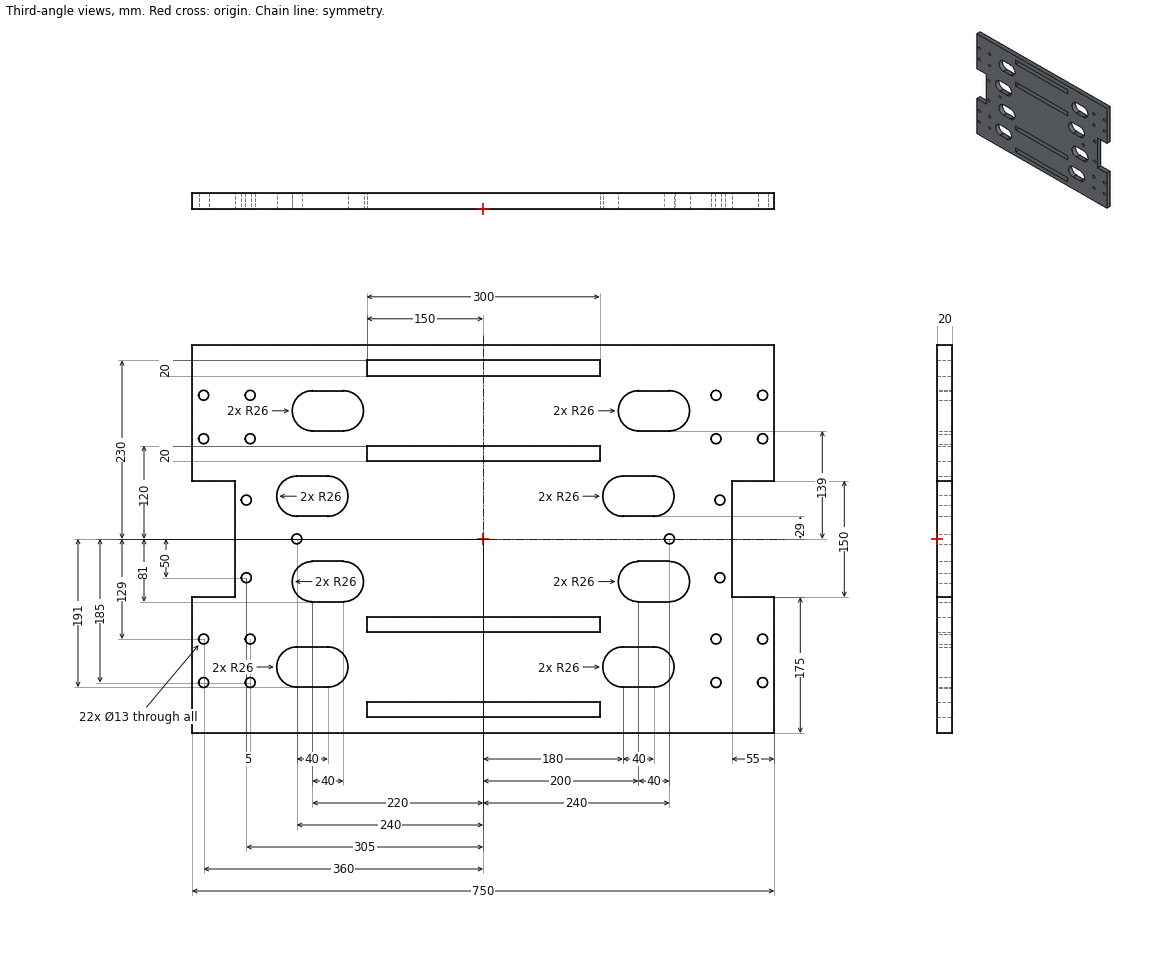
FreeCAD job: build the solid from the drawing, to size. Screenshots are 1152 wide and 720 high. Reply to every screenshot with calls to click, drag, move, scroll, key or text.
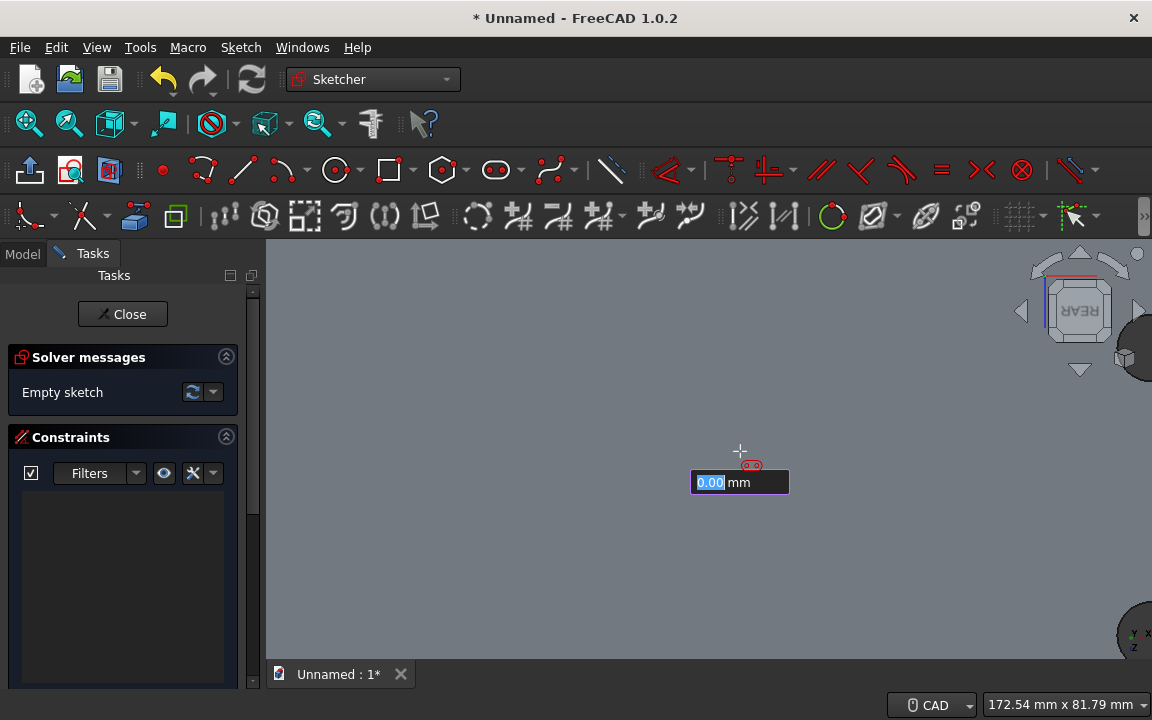
click(637, 317)
key(Escape)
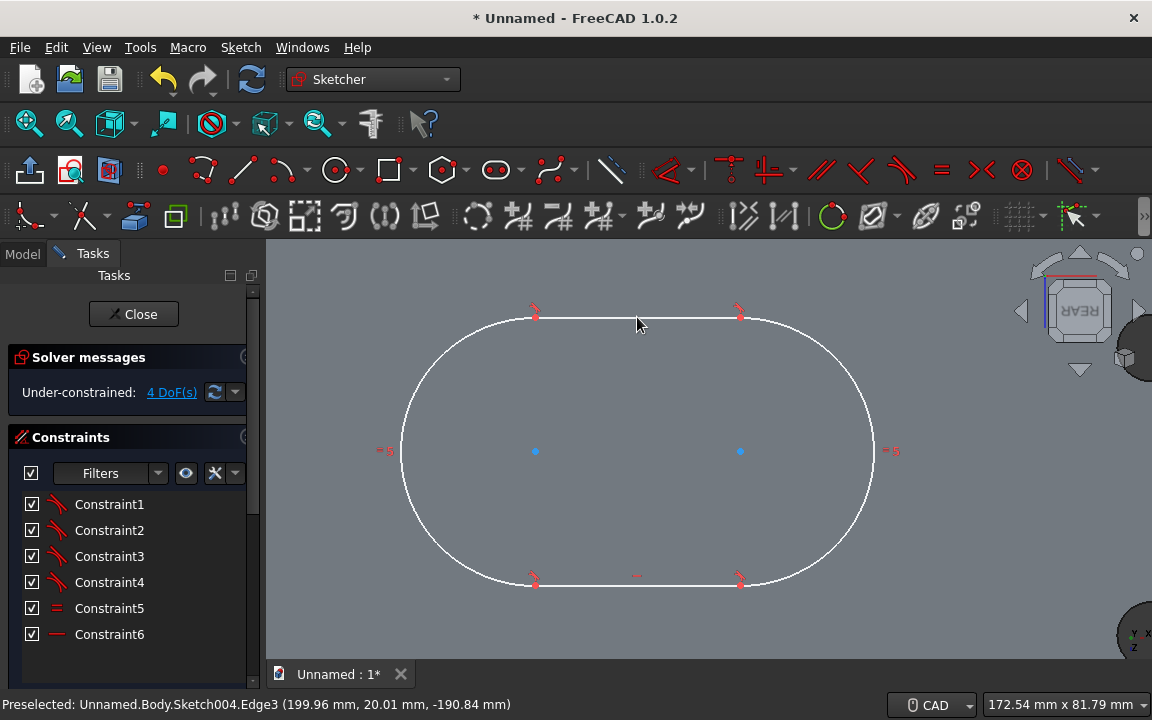
click(666, 170)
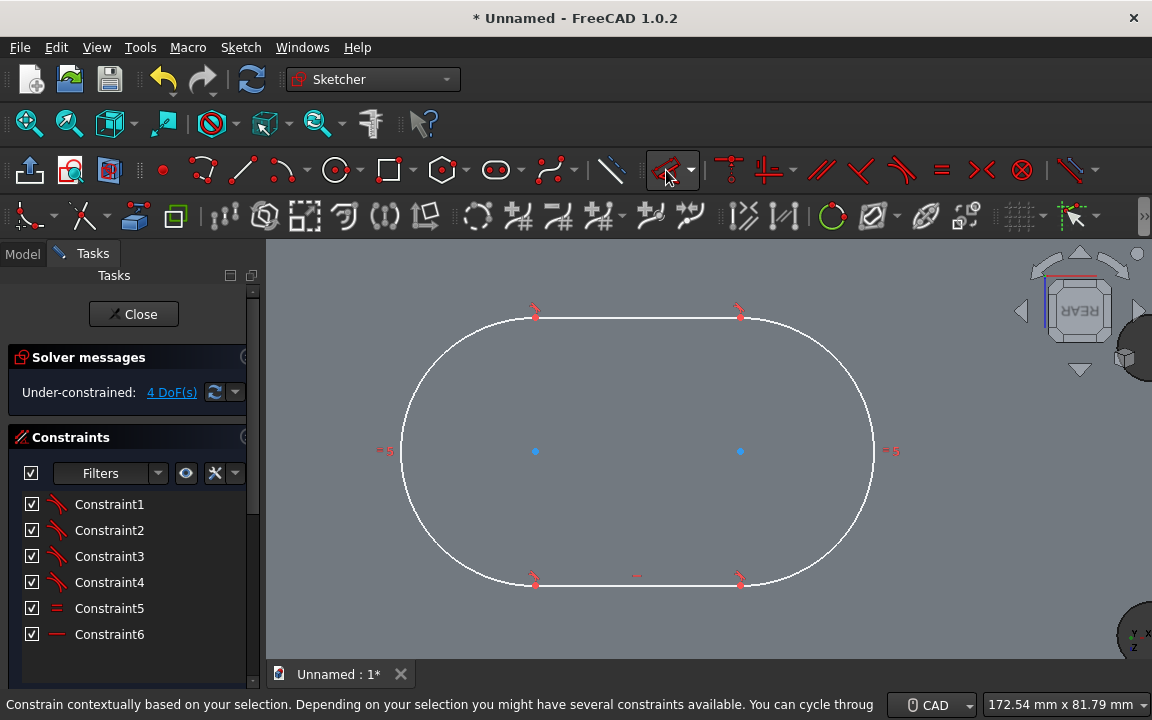
click(427, 373)
click(401, 354)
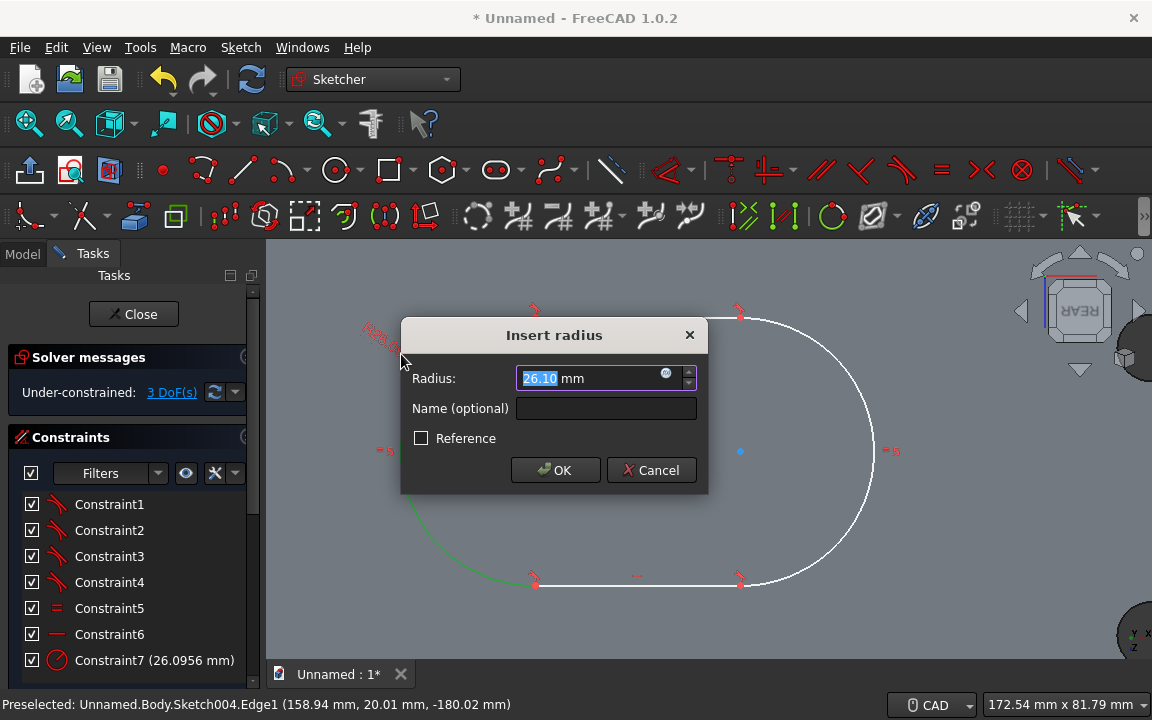
text(26)
key(Return)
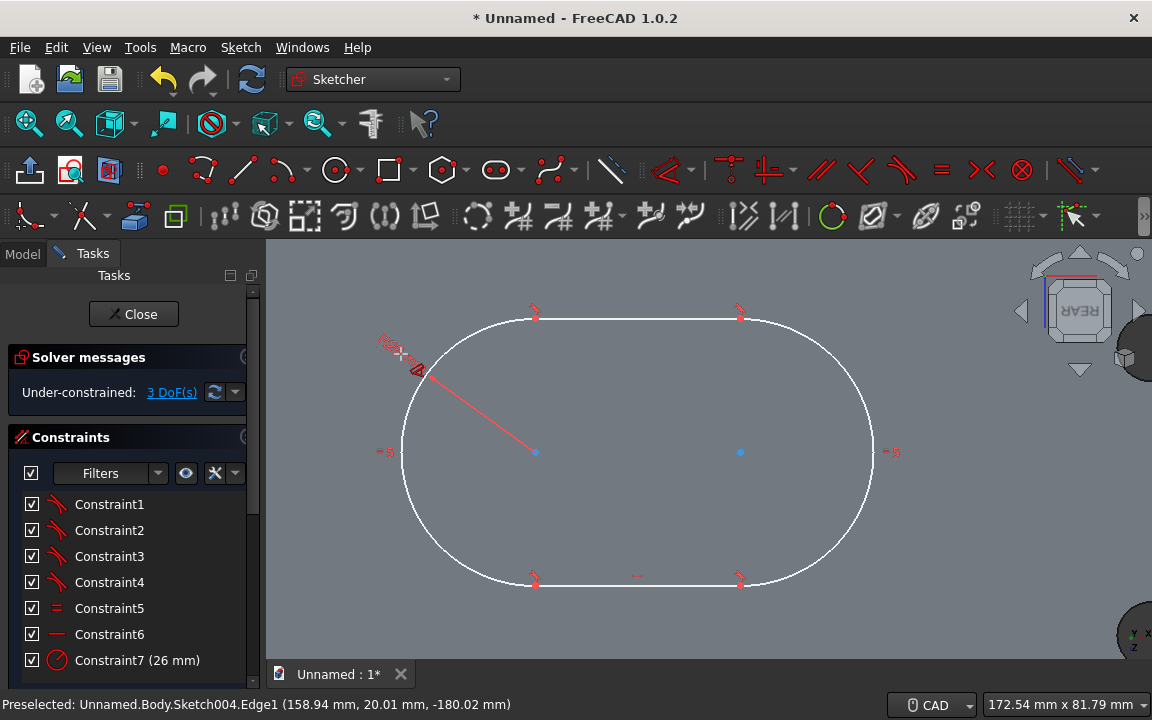
click(597, 319)
click(638, 285)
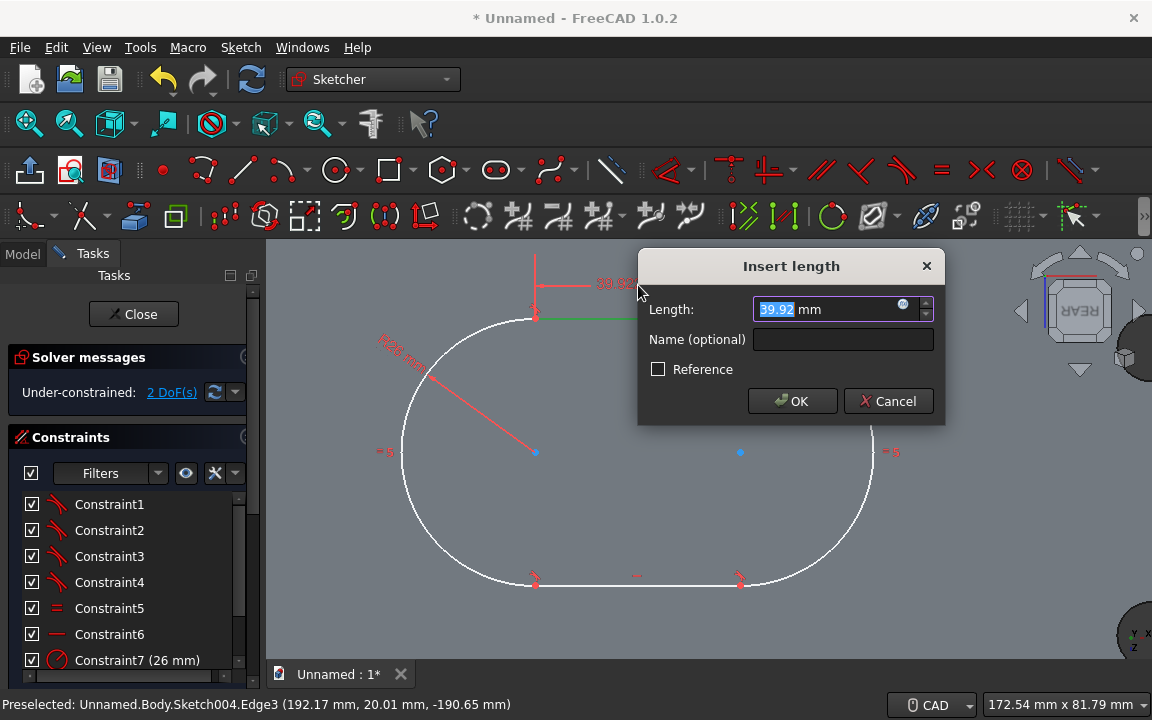
text(40)
key(Return)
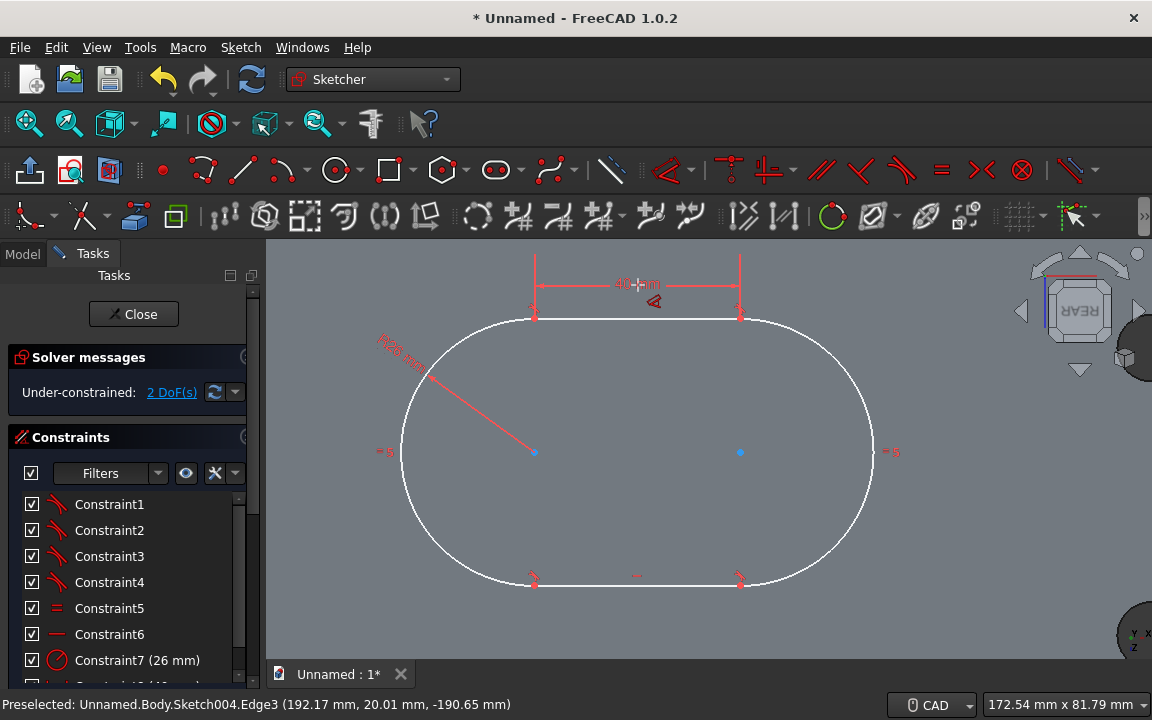
click(535, 319)
click(414, 285)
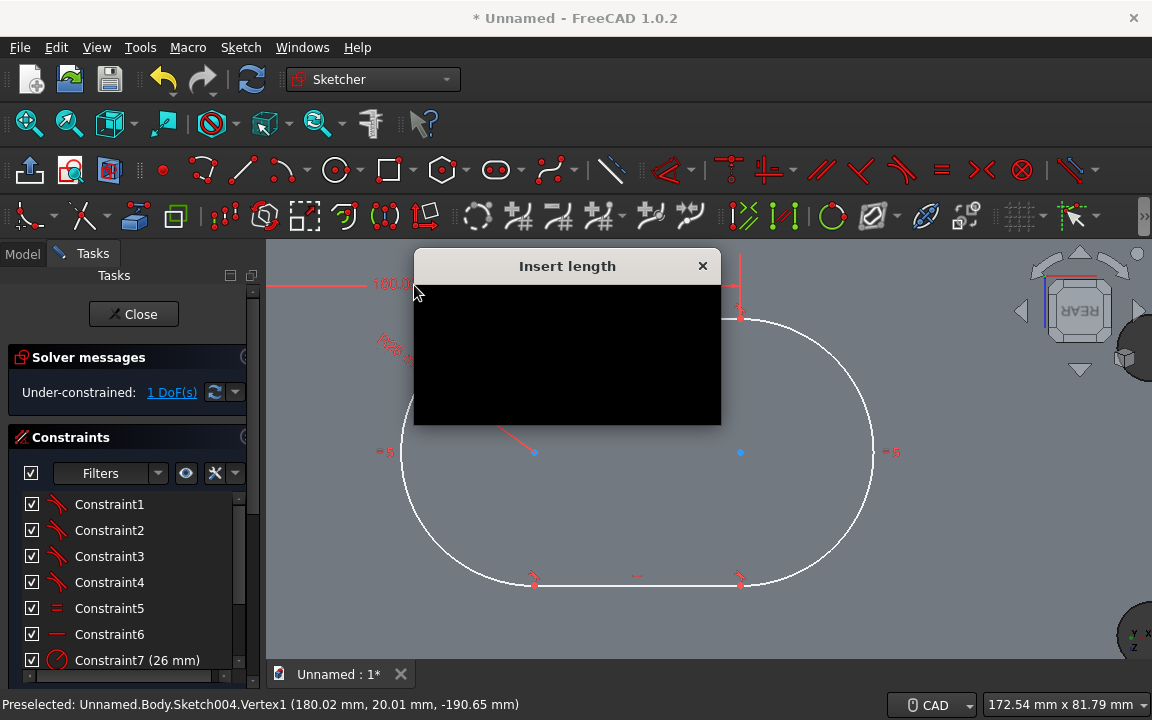
text(180)
key(Return)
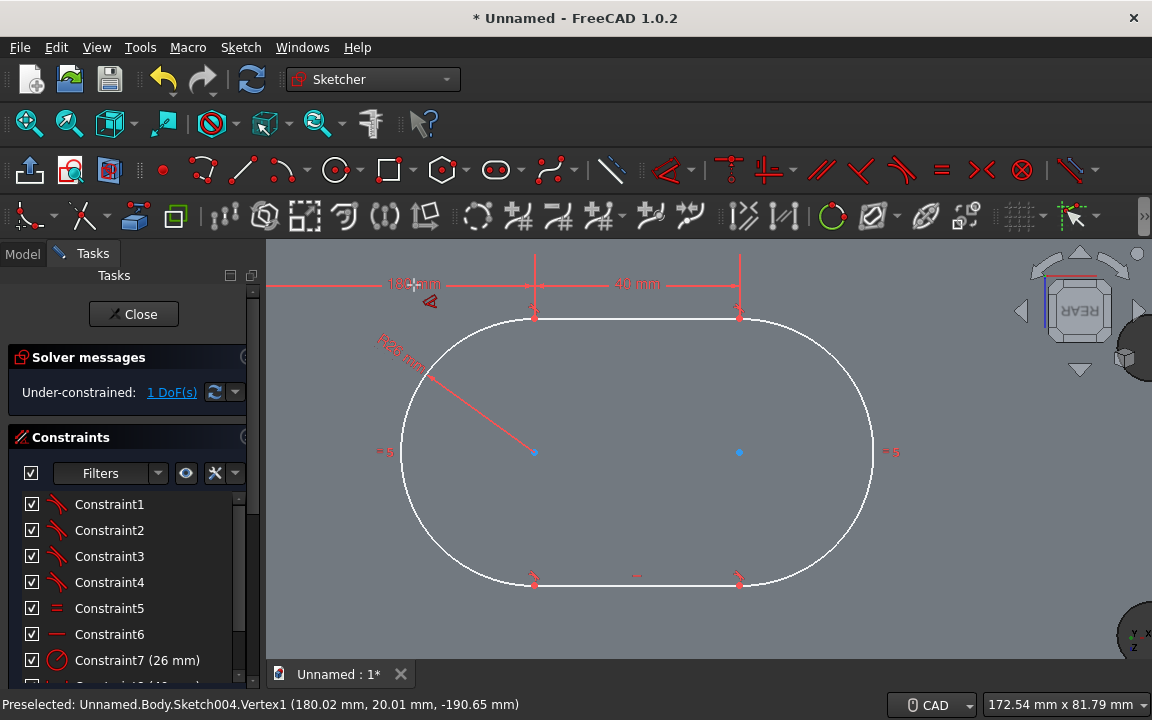
click(535, 319)
click(569, 475)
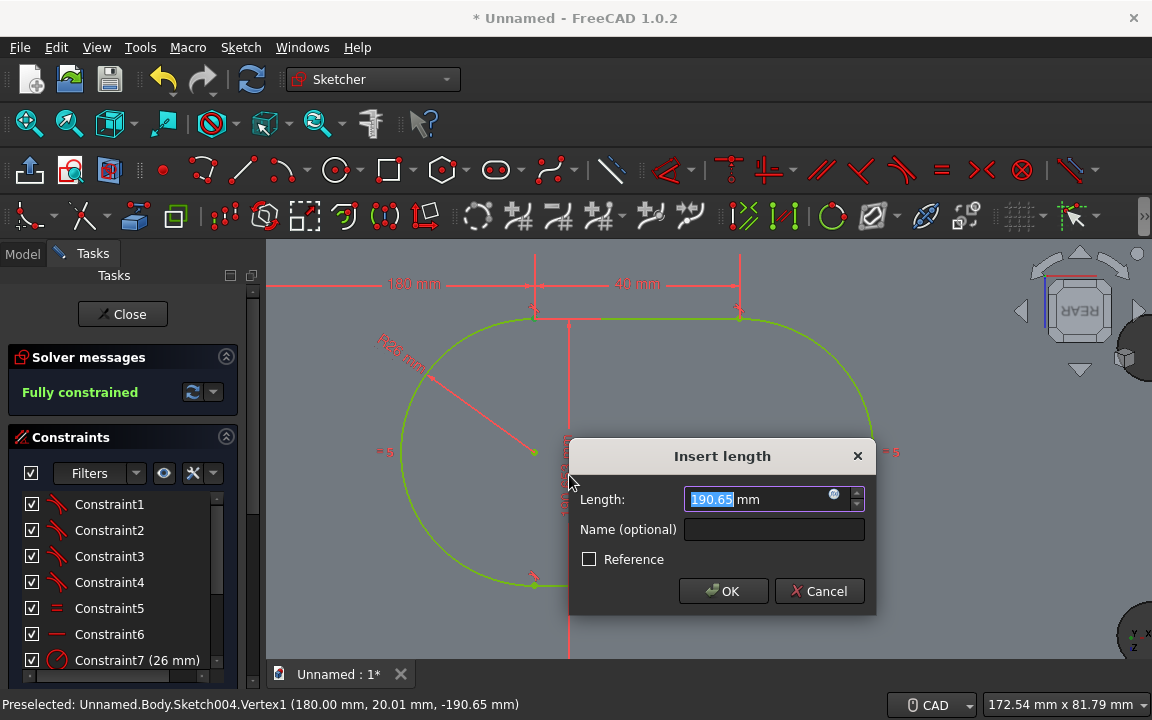
text(191)
key(Return)
key(Escape)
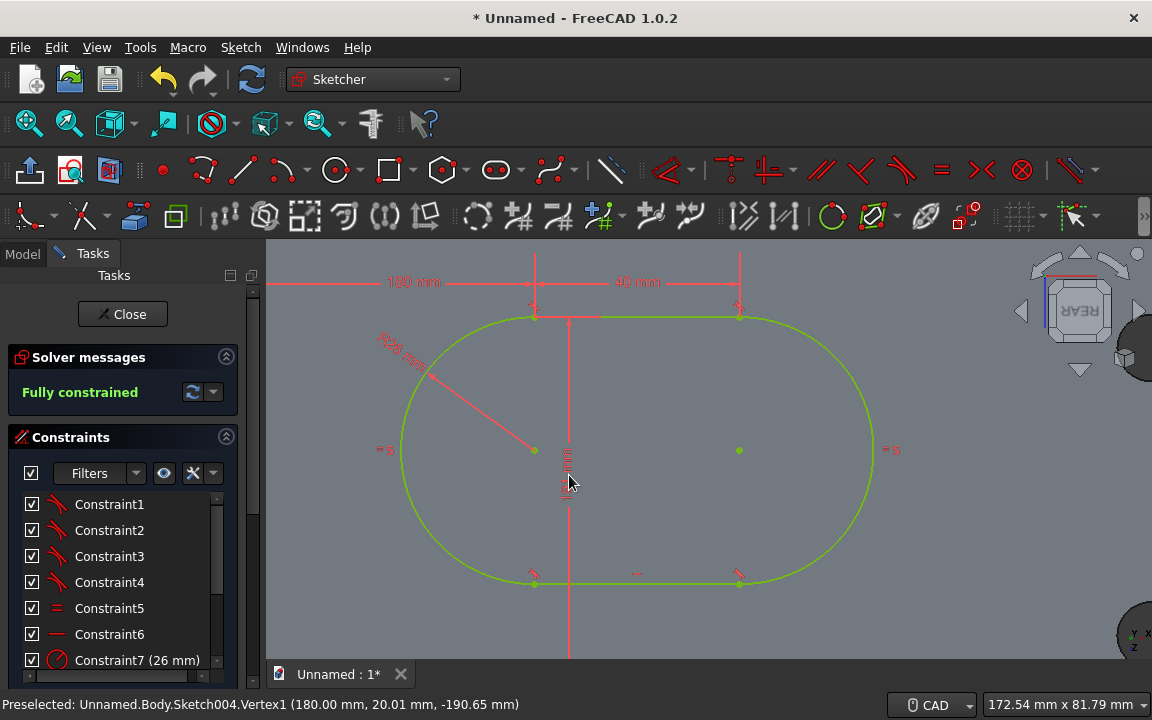
click(123, 314)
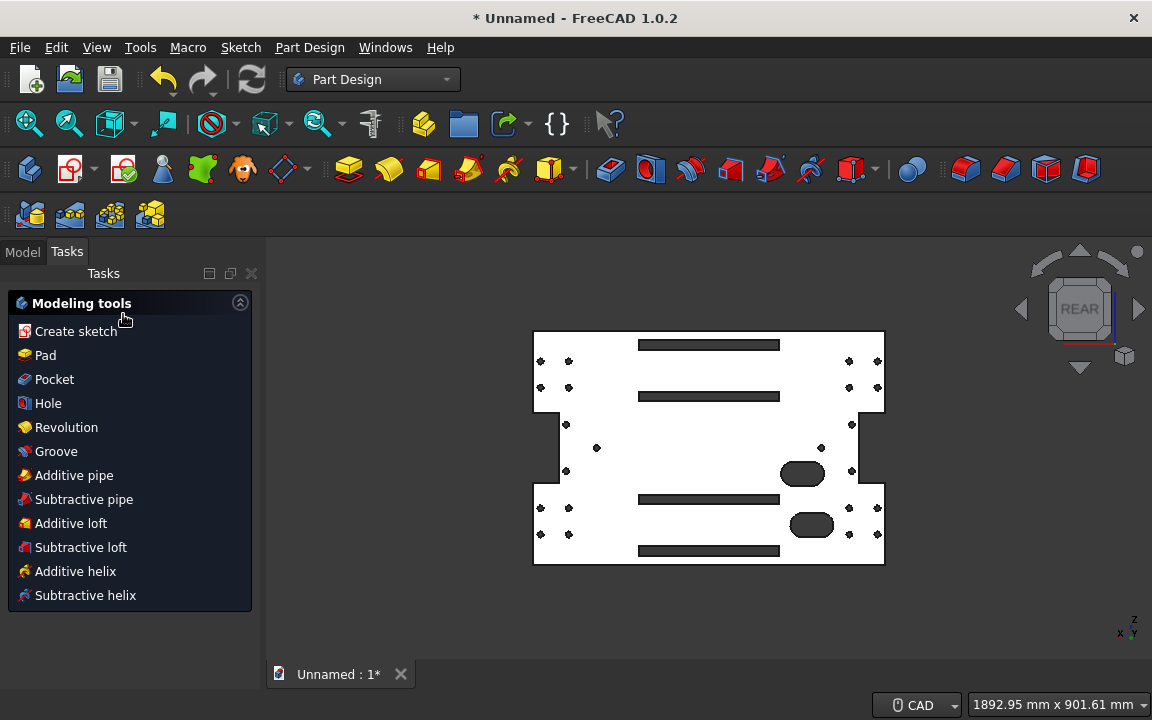
click(612, 170)